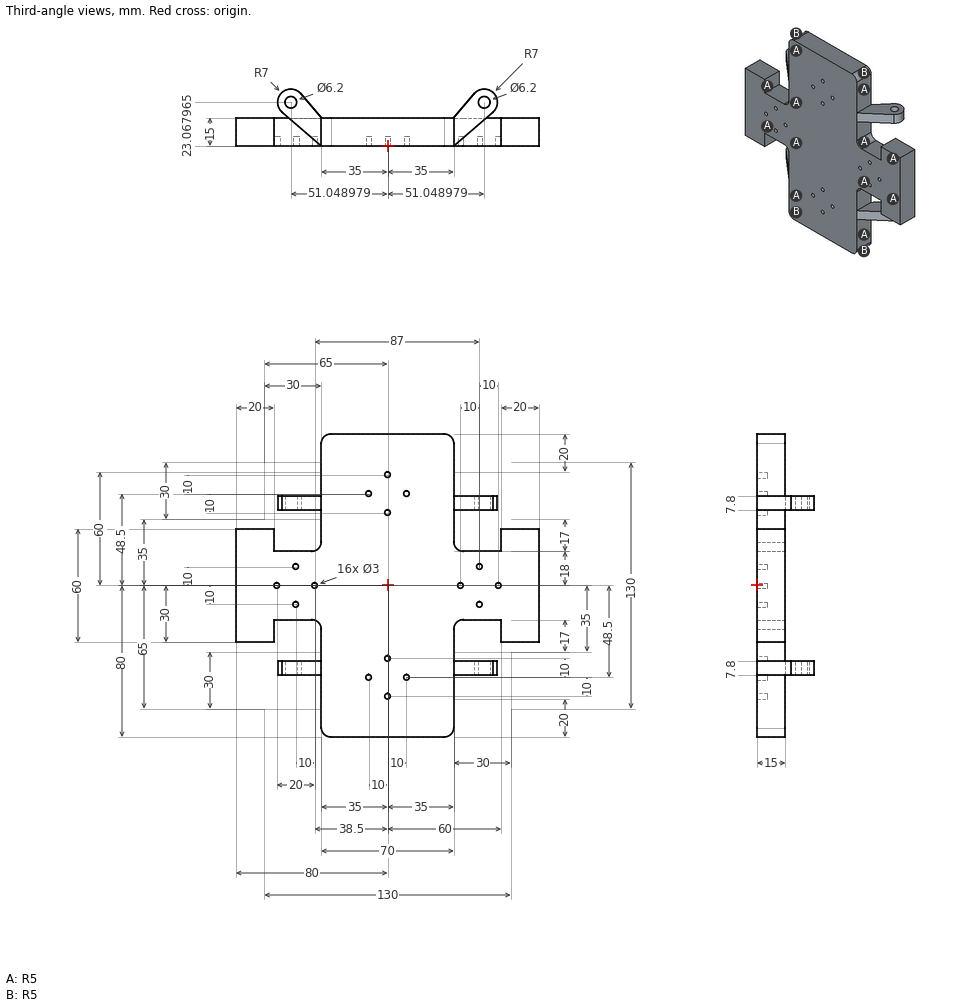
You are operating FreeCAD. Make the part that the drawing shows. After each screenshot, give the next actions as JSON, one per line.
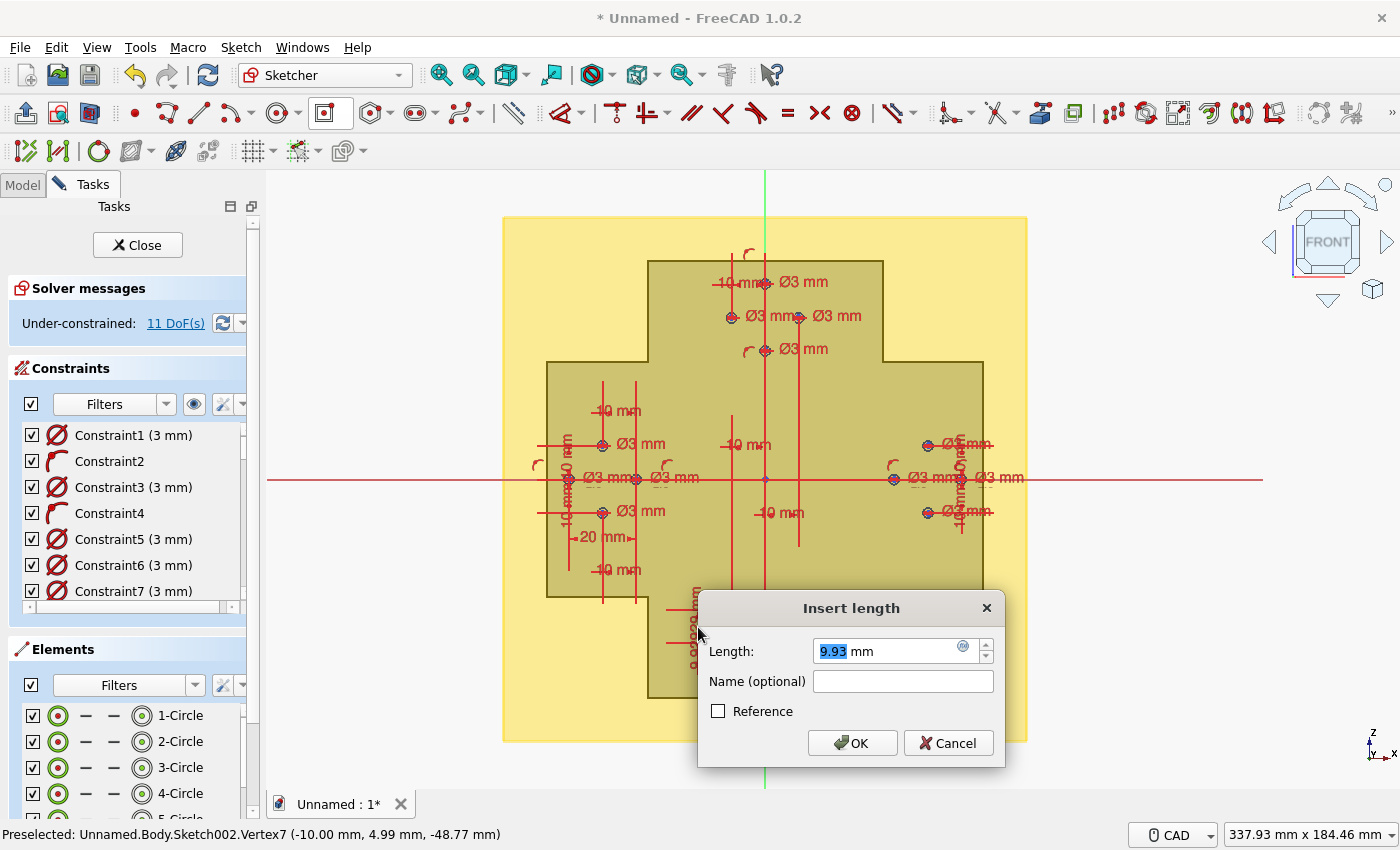
{"action": "type", "text": "10"}
{"action": "key", "text": "Return"}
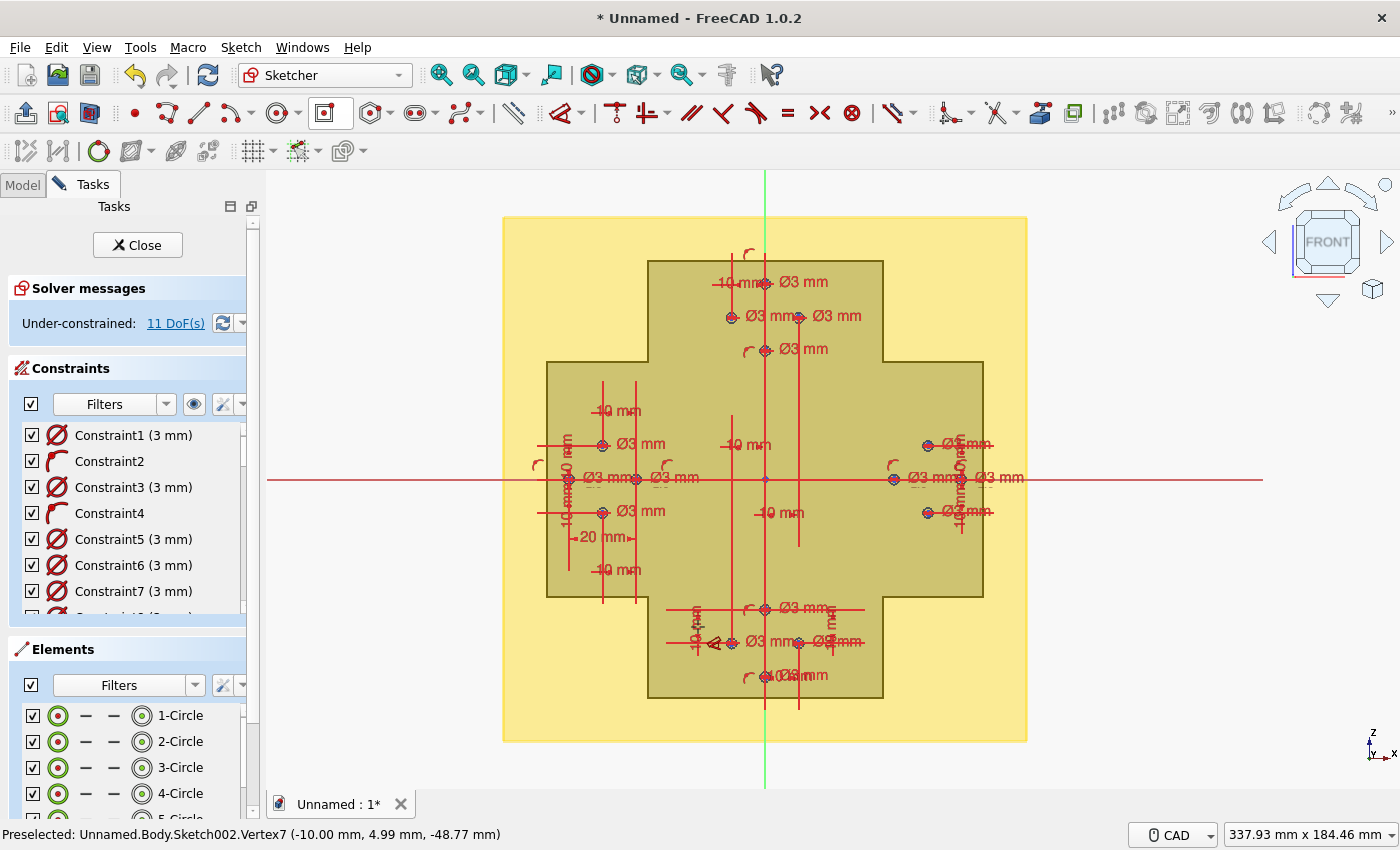
{"action": "left_click", "coordinate": [799, 643]}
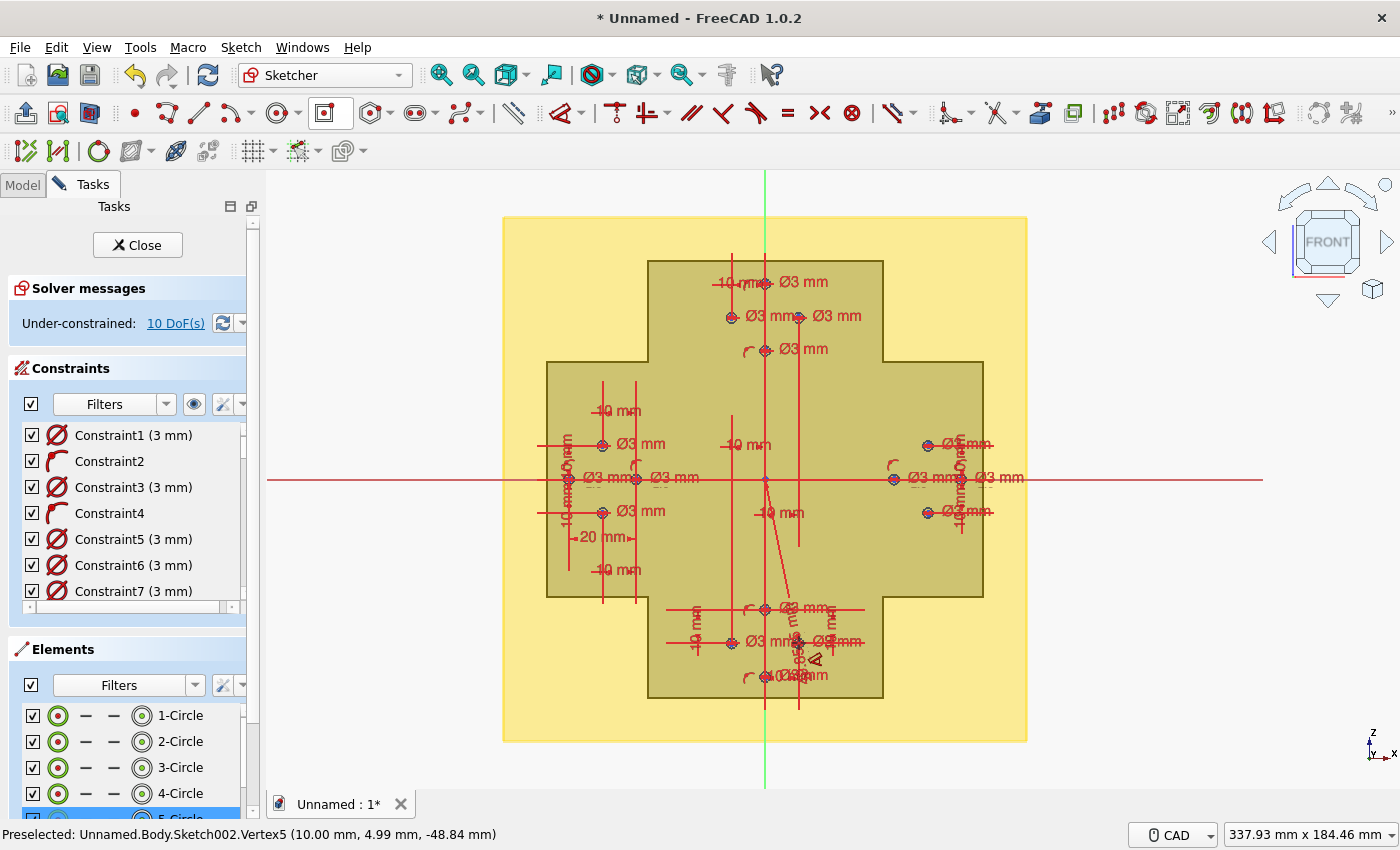
{"action": "left_click", "coordinate": [765, 677]}
{"action": "left_click", "coordinate": [833, 653]}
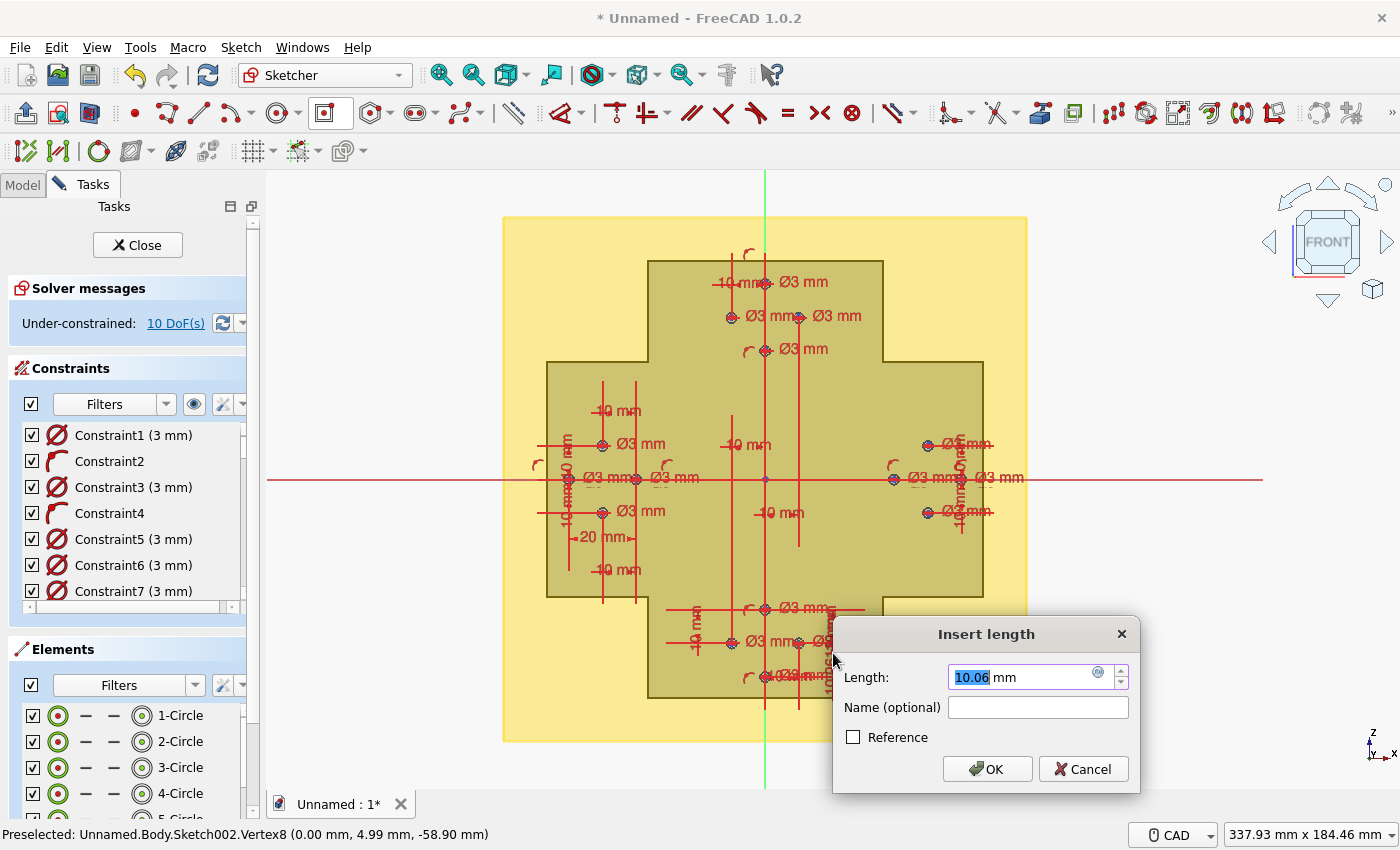
{"action": "type", "text": "10"}
{"action": "key", "text": "Return"}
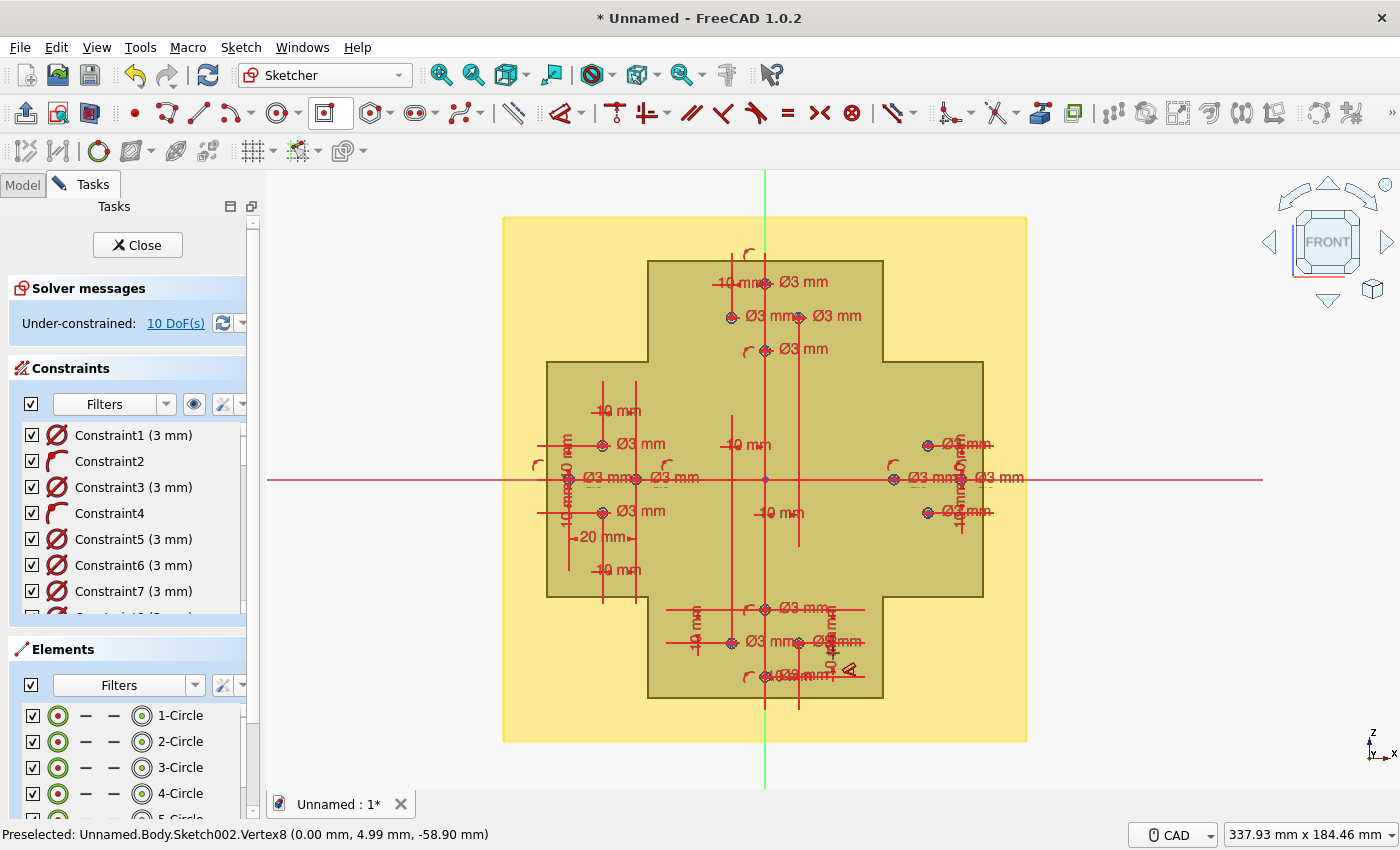
{"action": "left_click", "coordinate": [636, 480]}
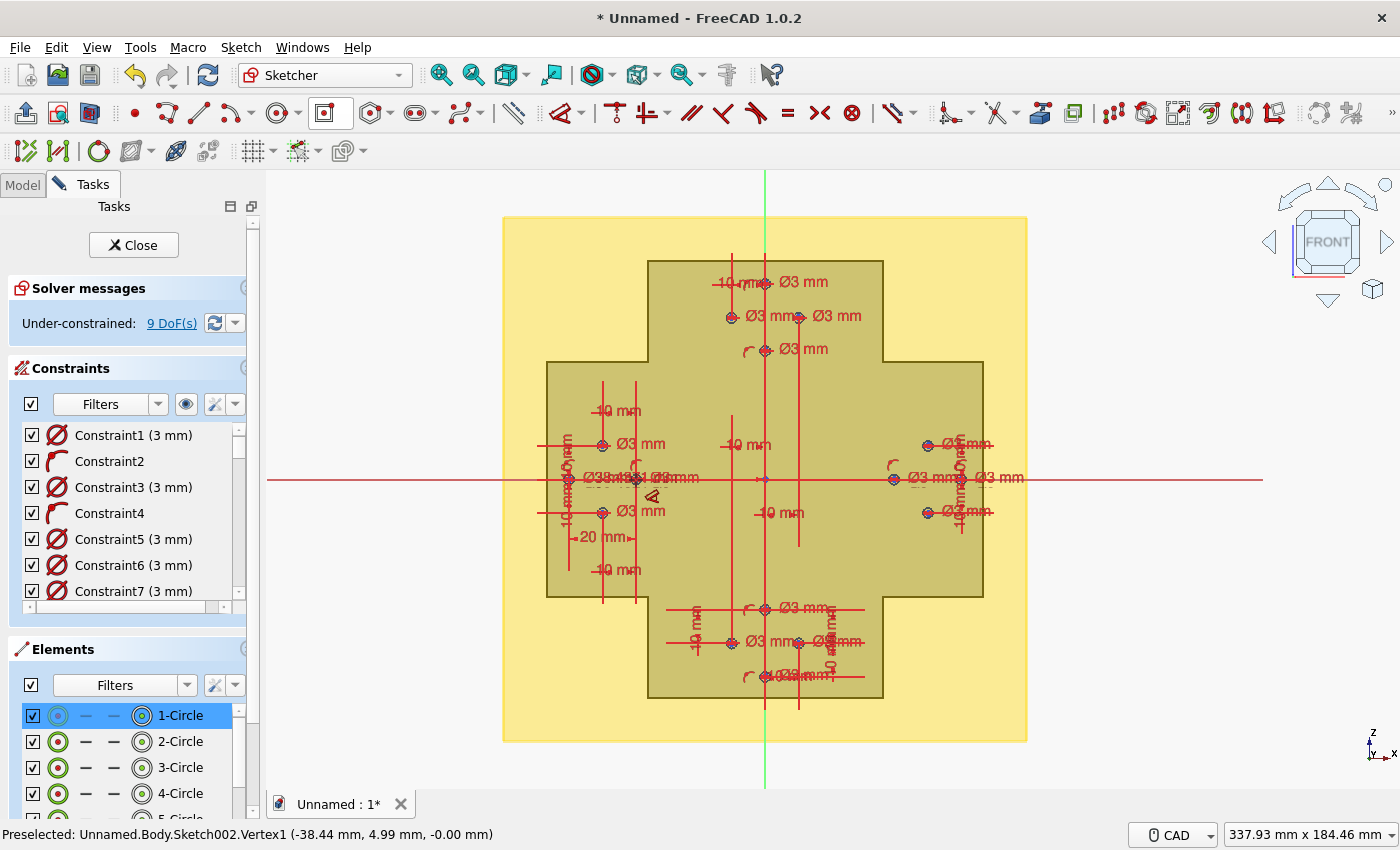
{"action": "left_click", "coordinate": [928, 446]}
{"action": "left_click", "coordinate": [782, 412]}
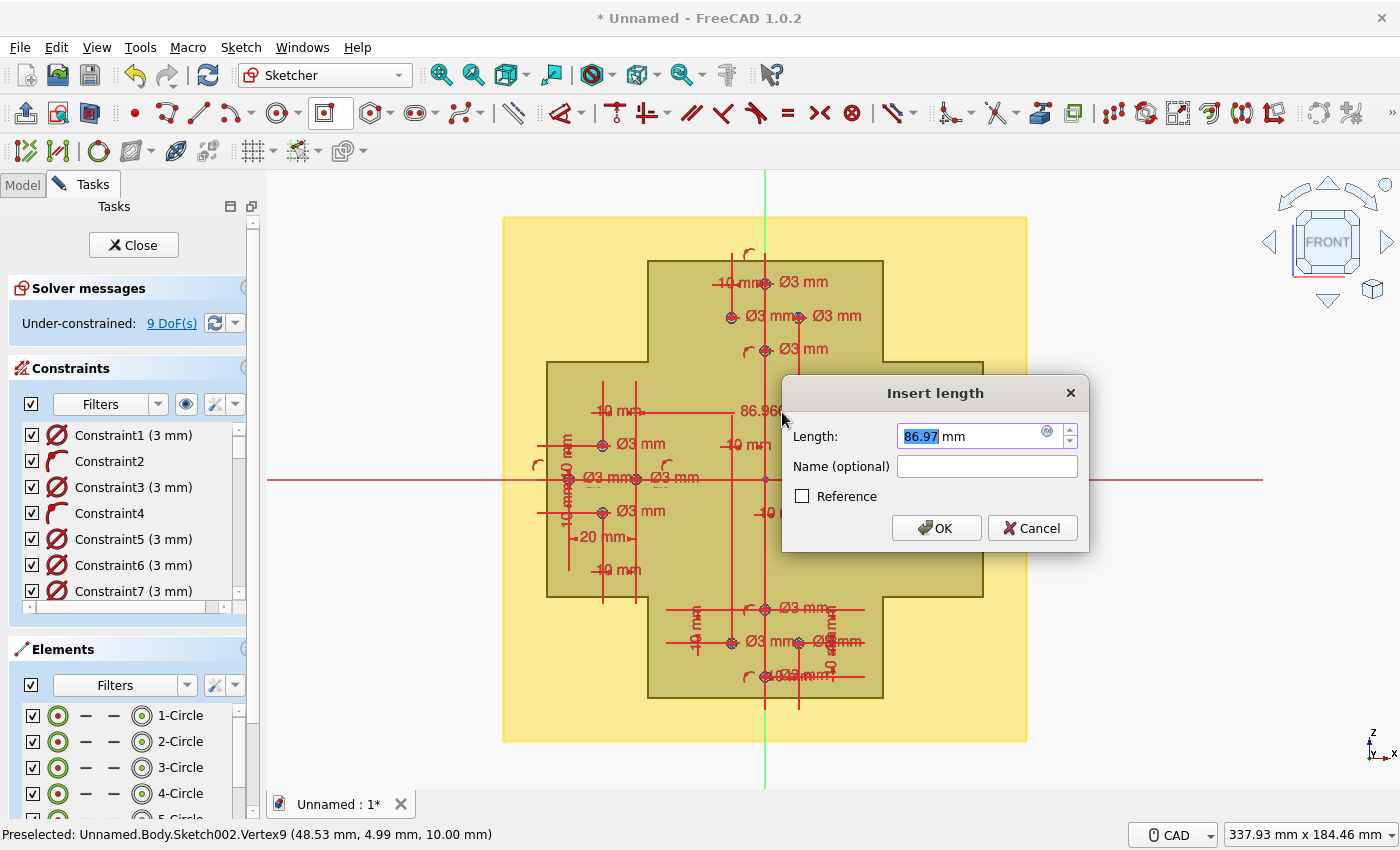
{"action": "type", "text": "87"}
{"action": "key", "text": "Return"}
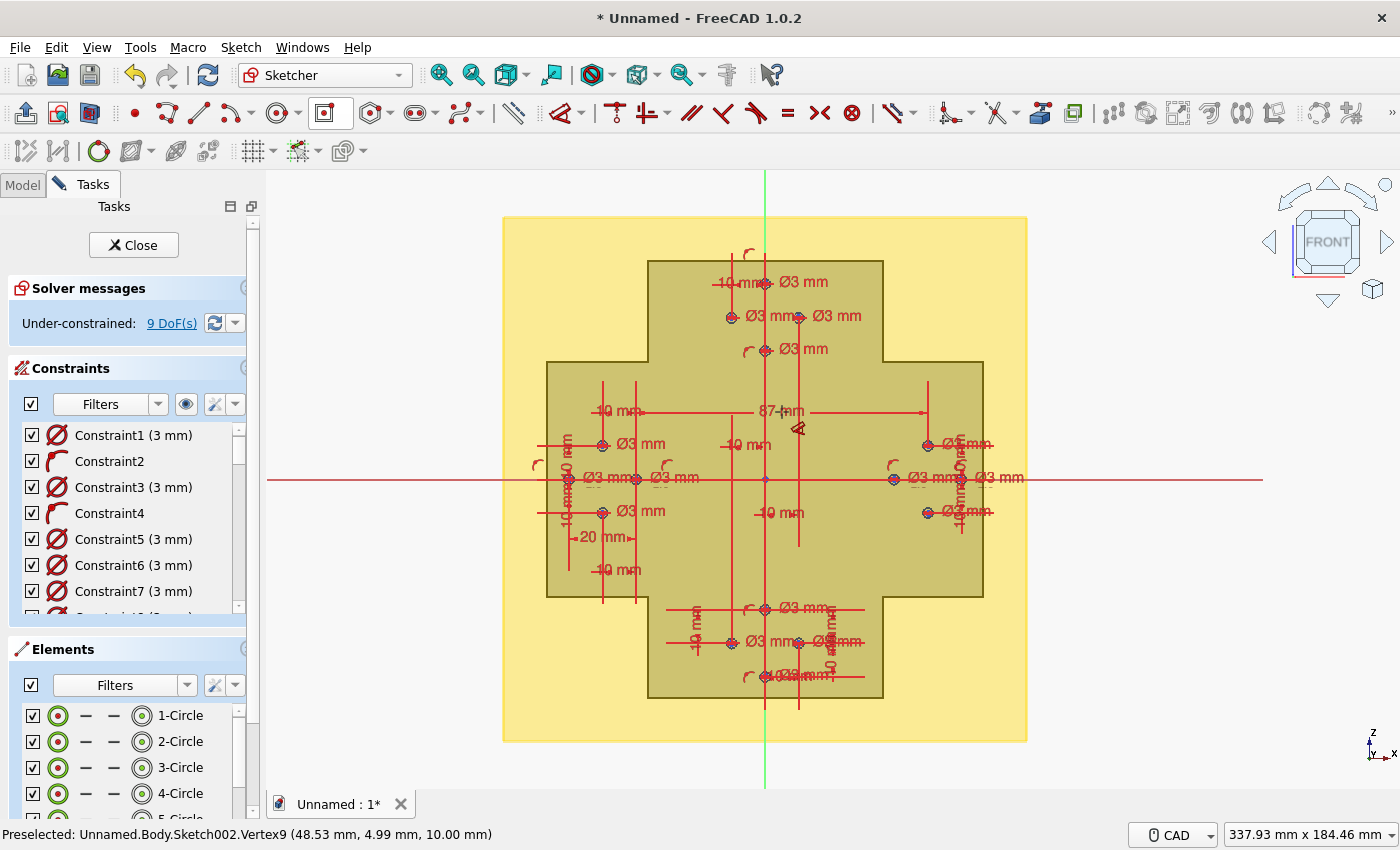
{"action": "left_click", "coordinate": [928, 446]}